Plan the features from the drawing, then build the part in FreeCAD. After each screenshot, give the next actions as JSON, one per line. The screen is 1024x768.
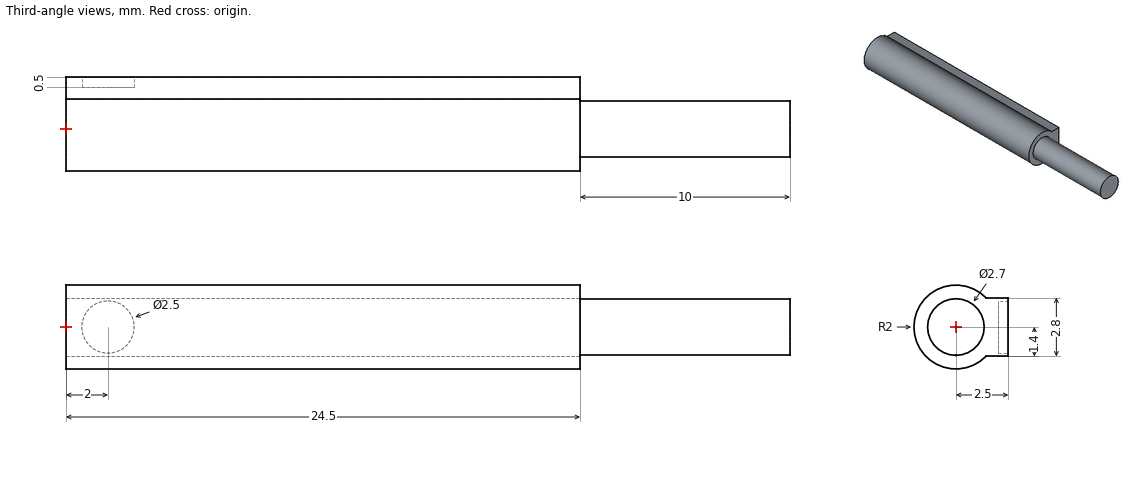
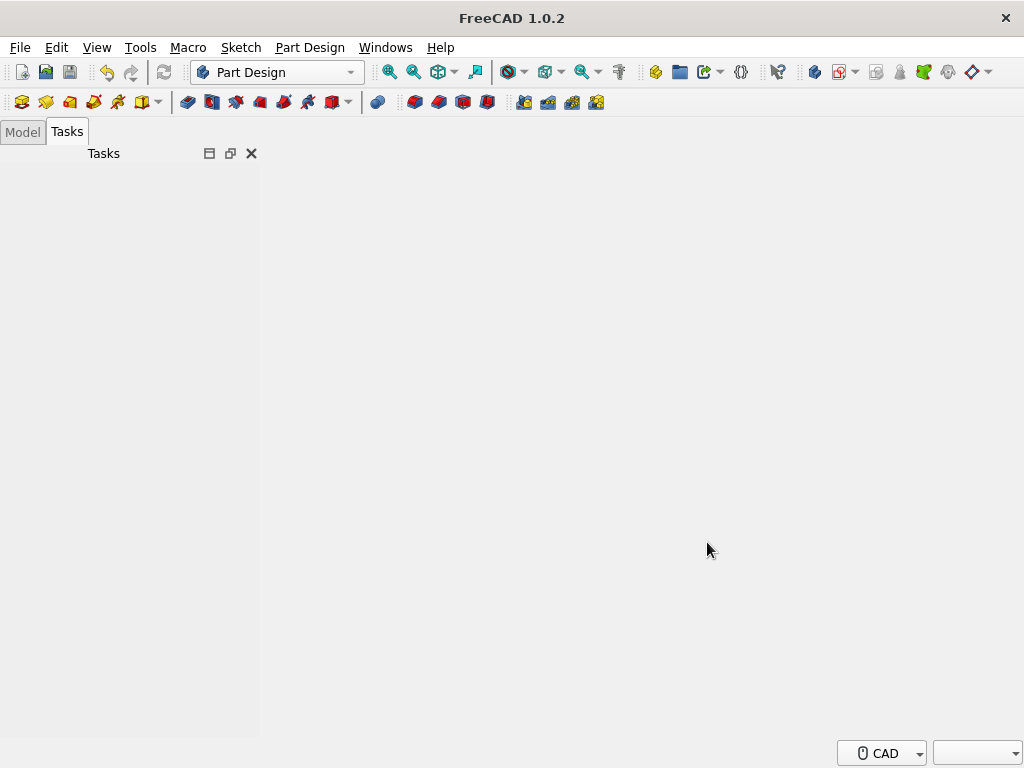
{"action": "key", "text": "ctrl+n"}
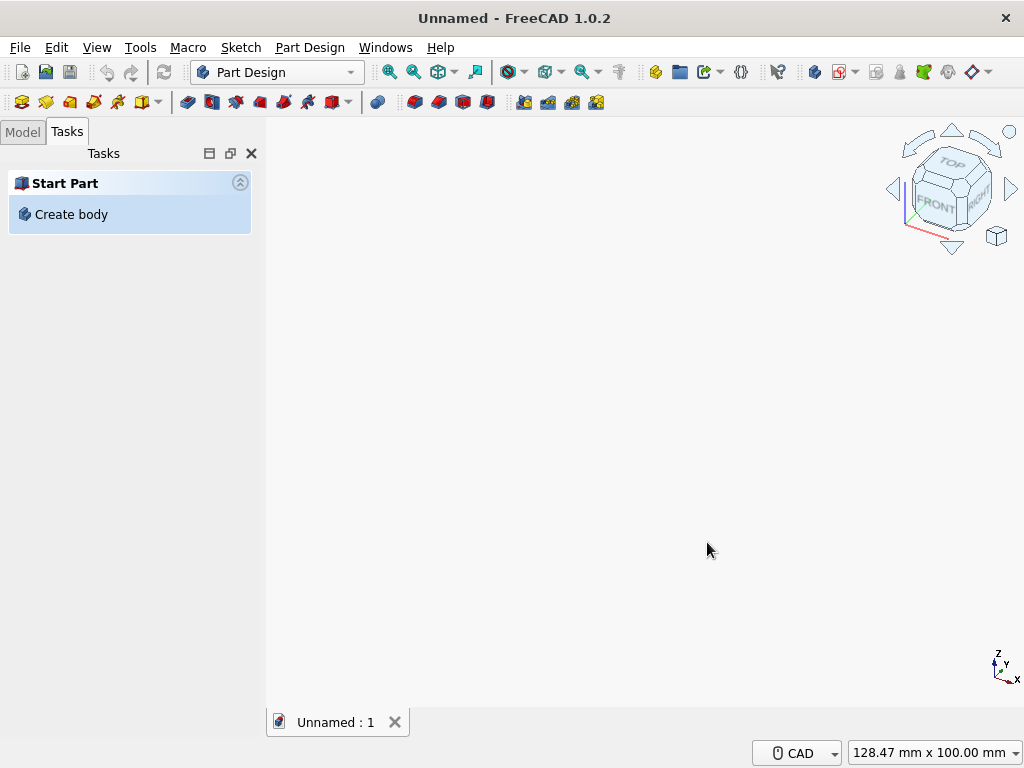
{"action": "left_click", "coordinate": [840, 72]}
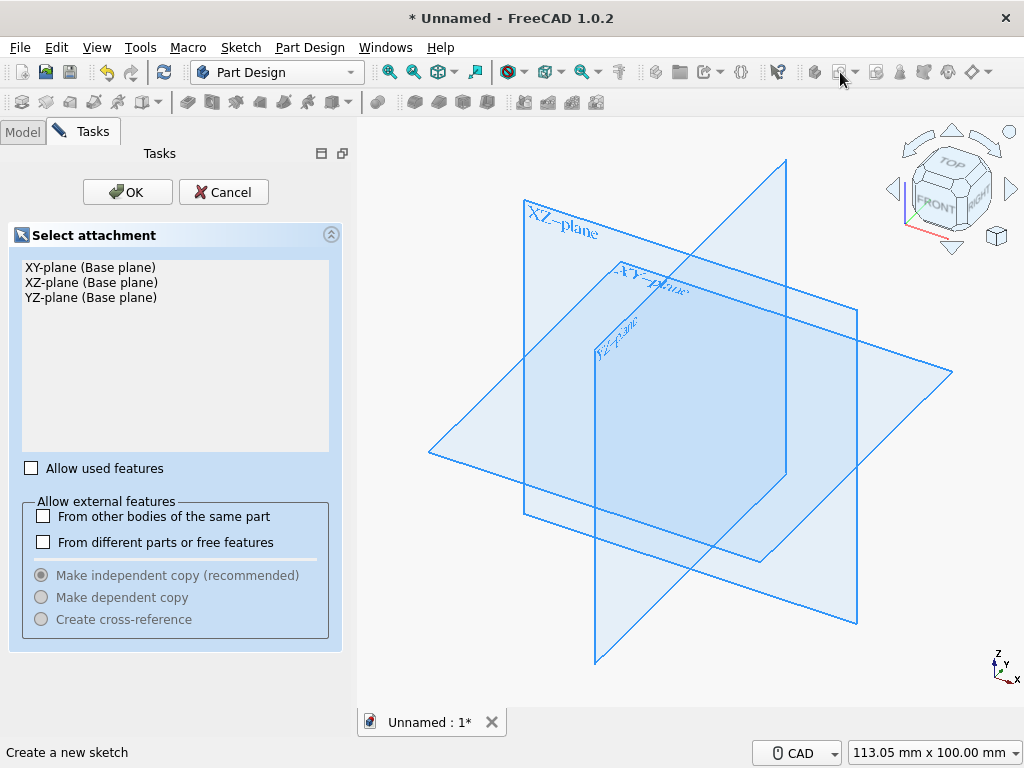
{"action": "left_click", "coordinate": [82, 298]}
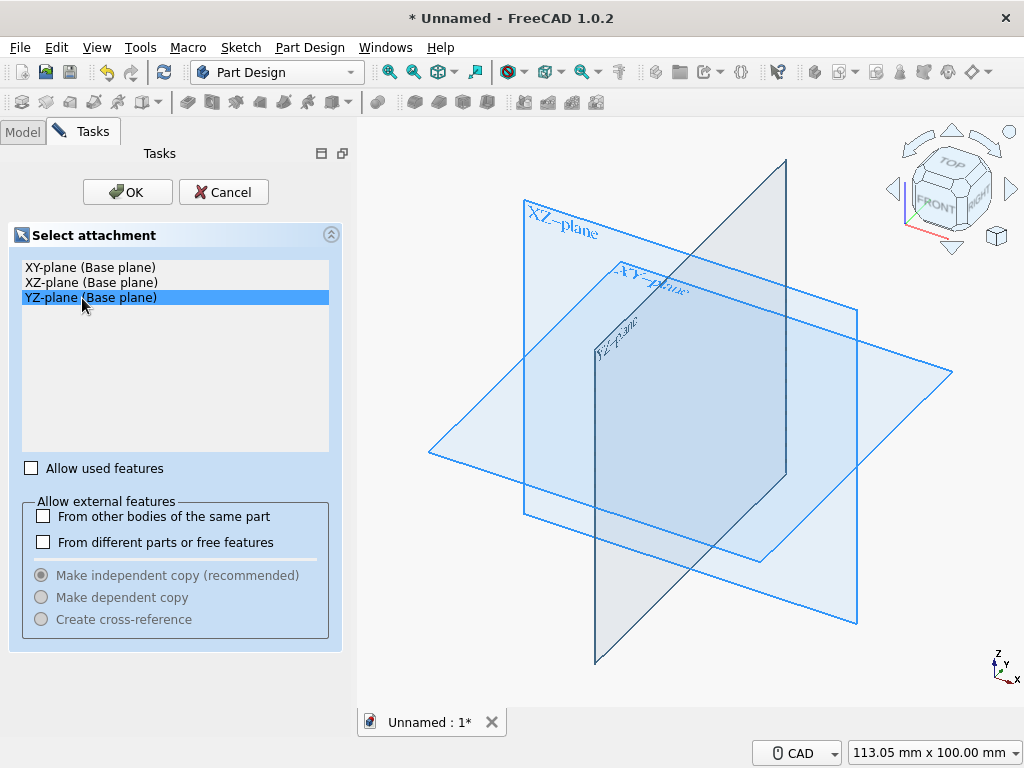
{"action": "left_click", "coordinate": [128, 192]}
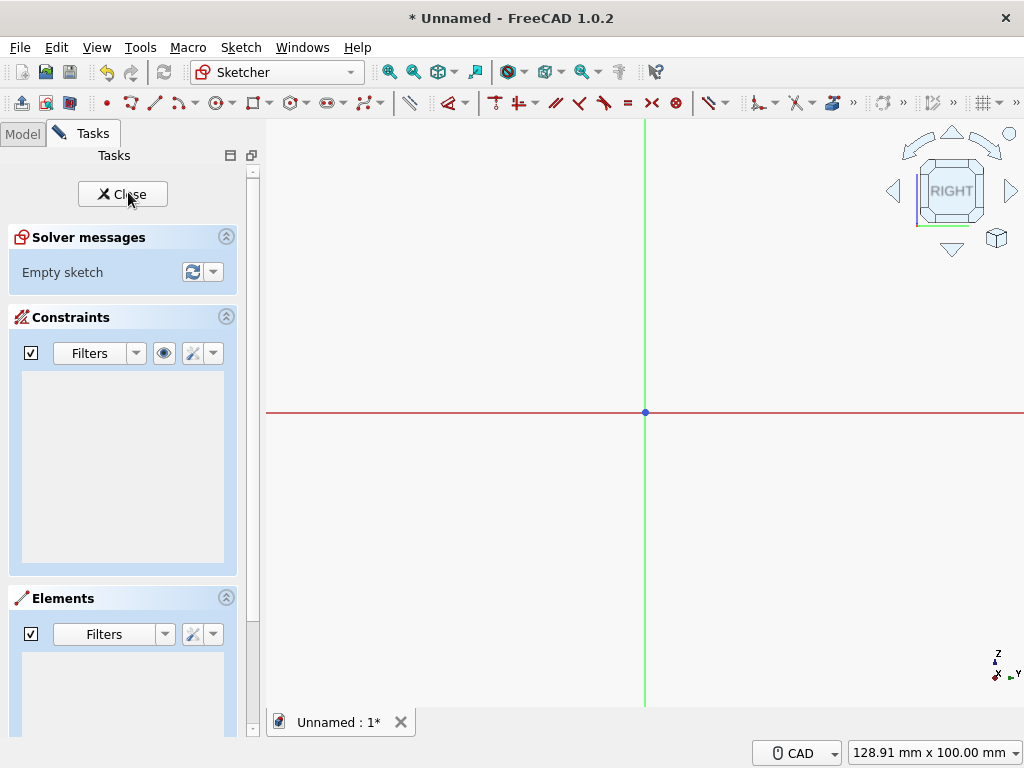
{"action": "scroll", "coordinate": [651, 413], "scroll_direction": "up", "scroll_amount": 14}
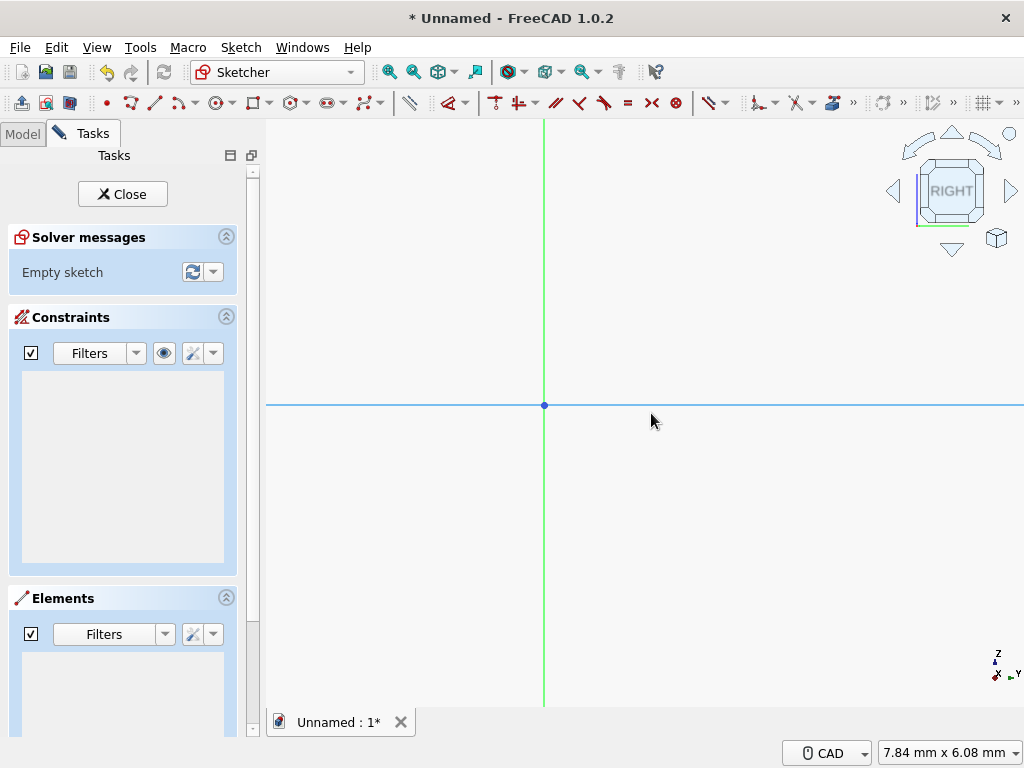
{"action": "key", "text": "g m"}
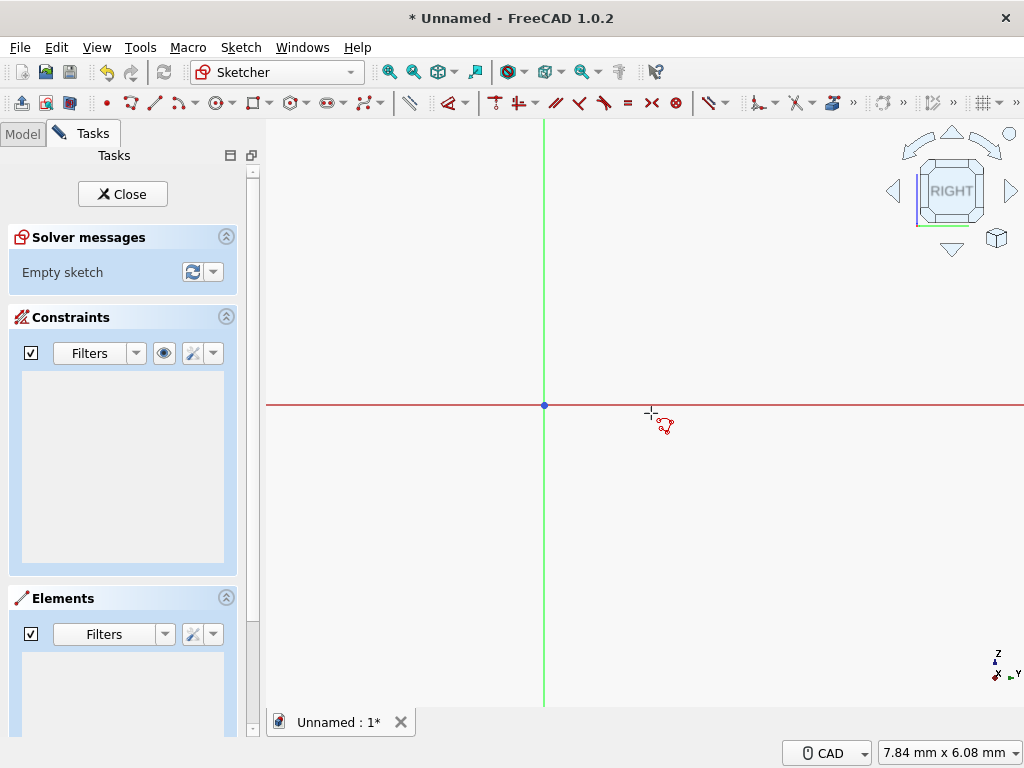
{"action": "left_click", "coordinate": [683, 541]}
{"action": "left_click", "coordinate": [786, 541]}
{"action": "left_click", "coordinate": [786, 270]}
{"action": "left_click", "coordinate": [683, 270]}
{"action": "right_click", "coordinate": [683, 270]}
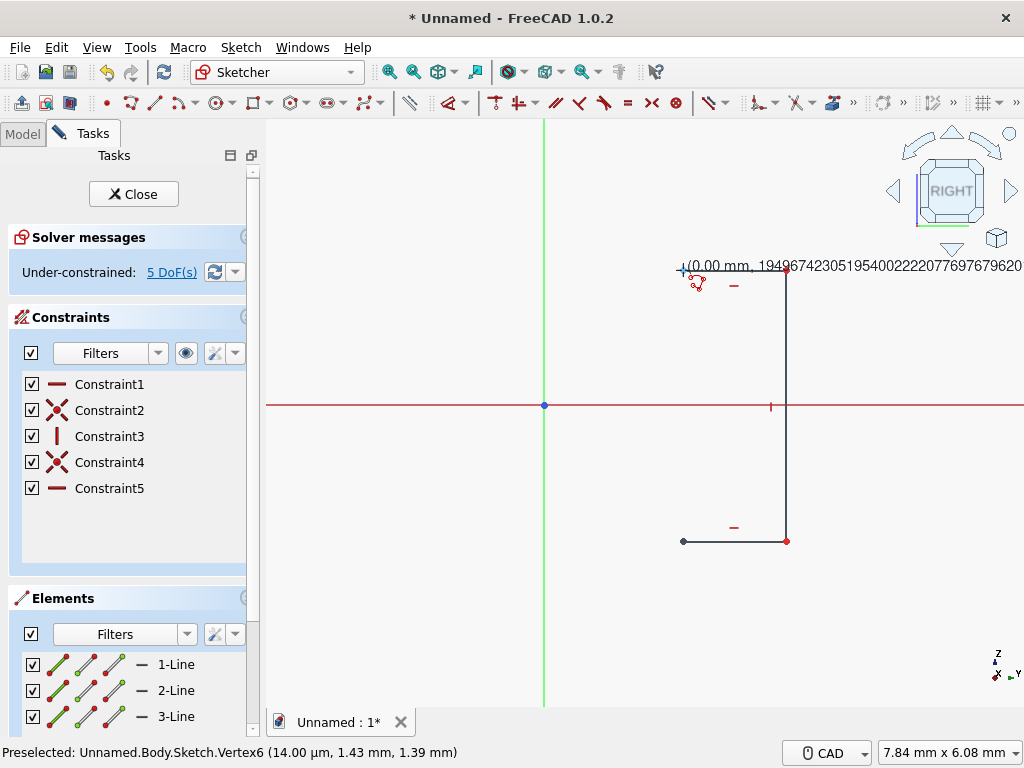
{"action": "key", "text": "g 3 a"}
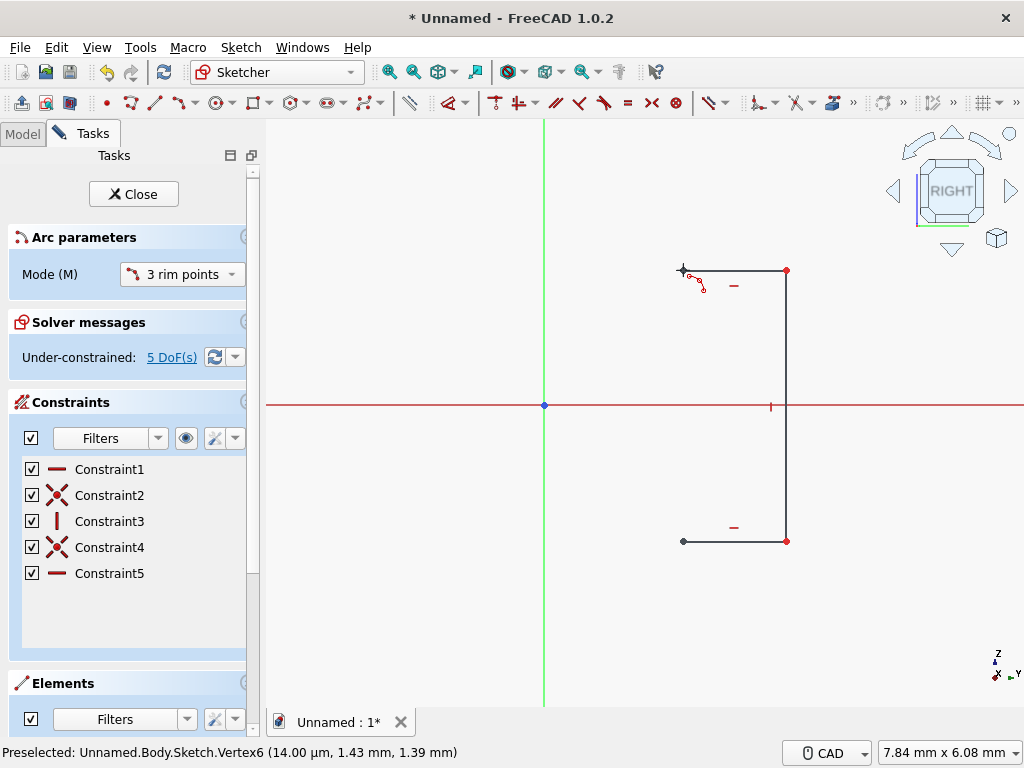
{"action": "left_click", "coordinate": [683, 271]}
{"action": "left_click", "coordinate": [683, 542]}
{"action": "left_click", "coordinate": [372, 317]}
{"action": "key", "text": "Escape"}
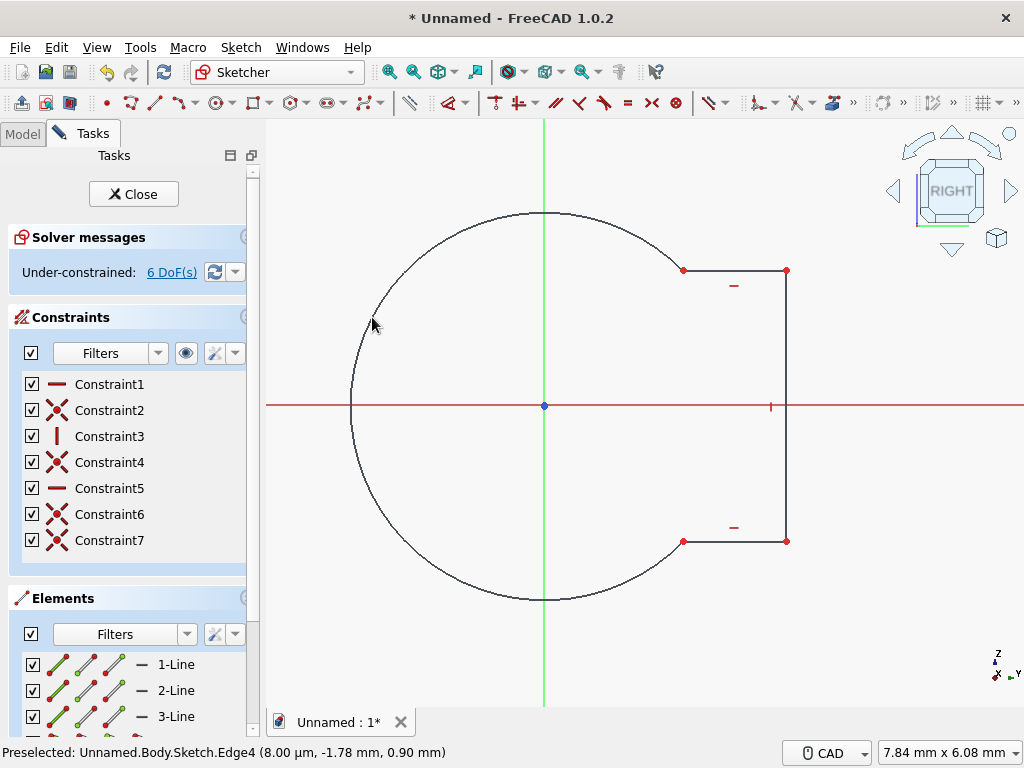
{"action": "left_click_drag", "start_coordinate": [534, 395], "coordinate": [554, 416]}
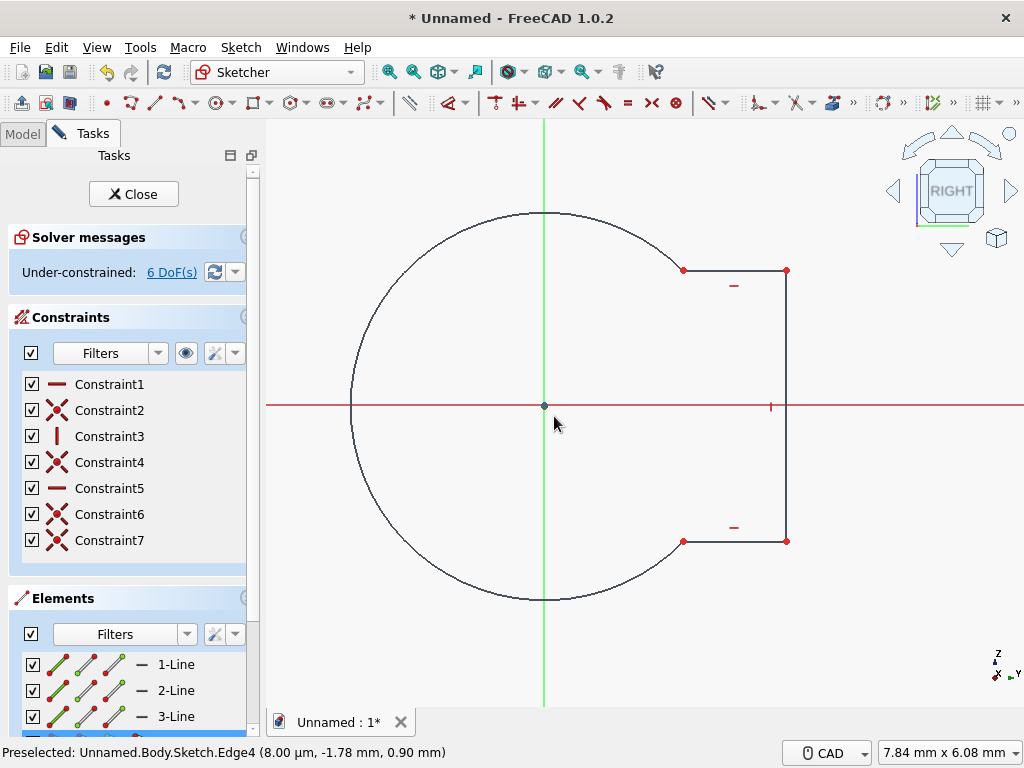
{"action": "key", "text": "c"}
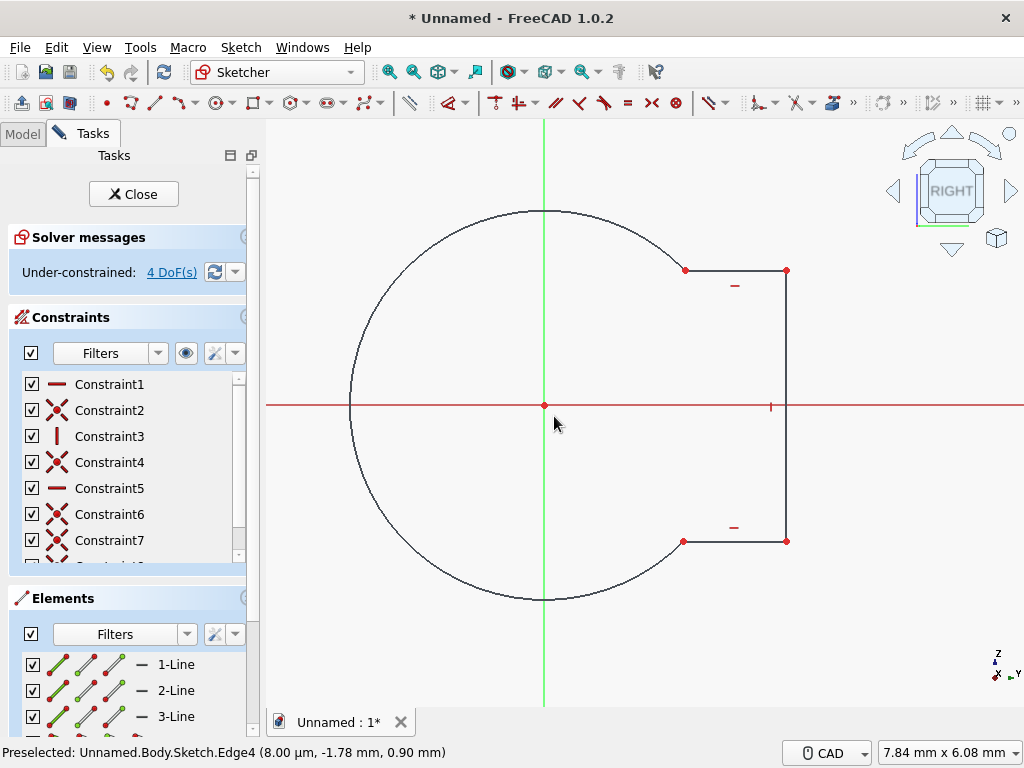
{"action": "left_click", "coordinate": [432, 246]}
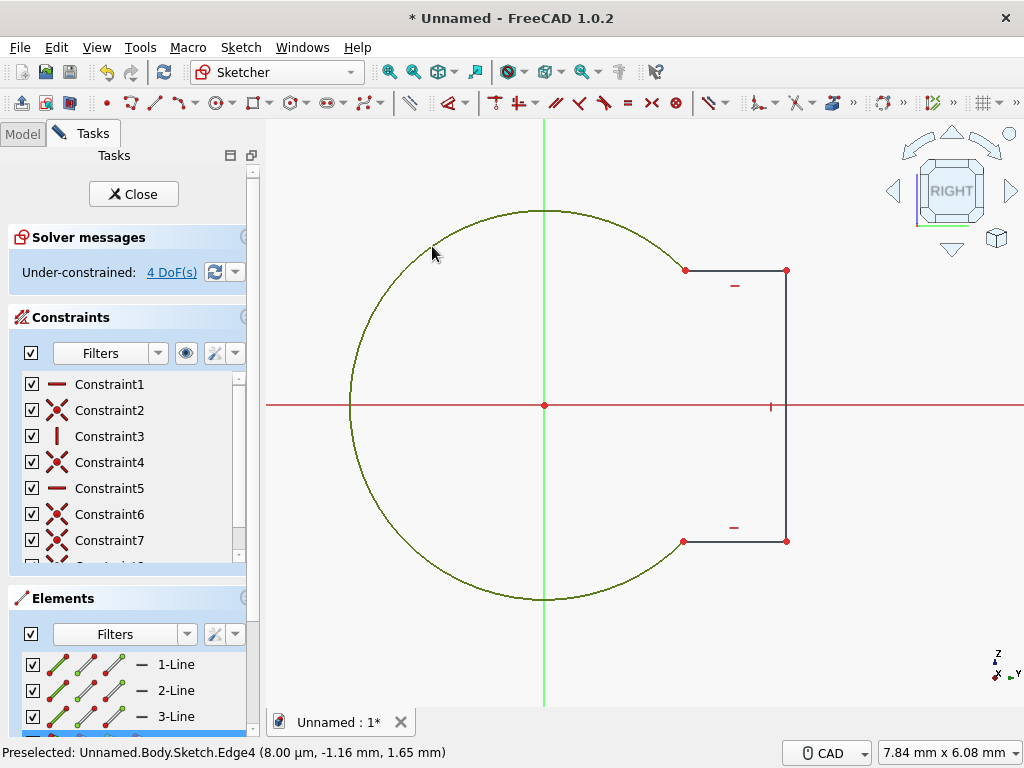
{"action": "key", "text": "k r"}